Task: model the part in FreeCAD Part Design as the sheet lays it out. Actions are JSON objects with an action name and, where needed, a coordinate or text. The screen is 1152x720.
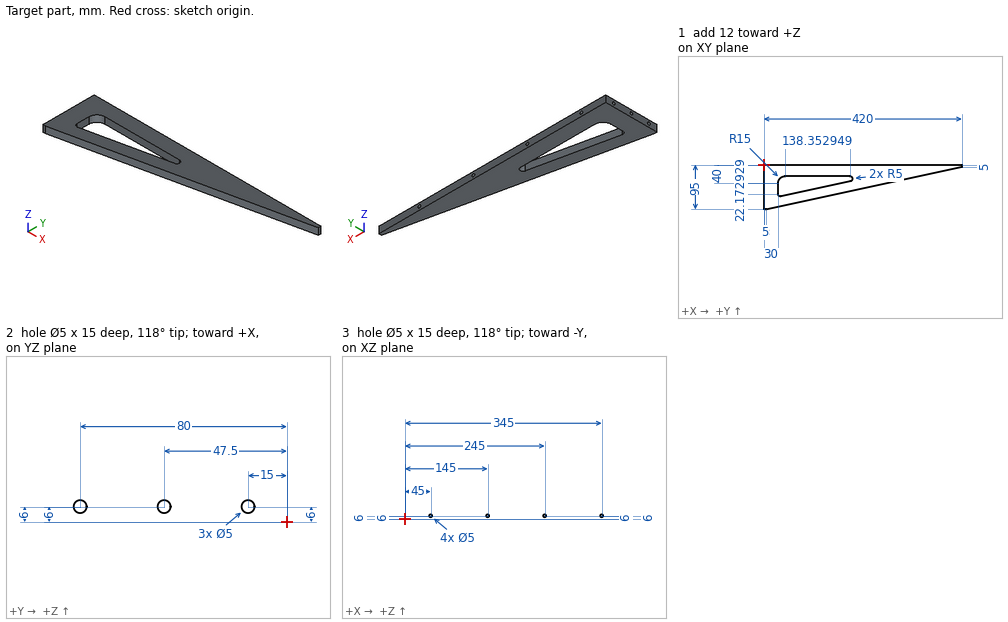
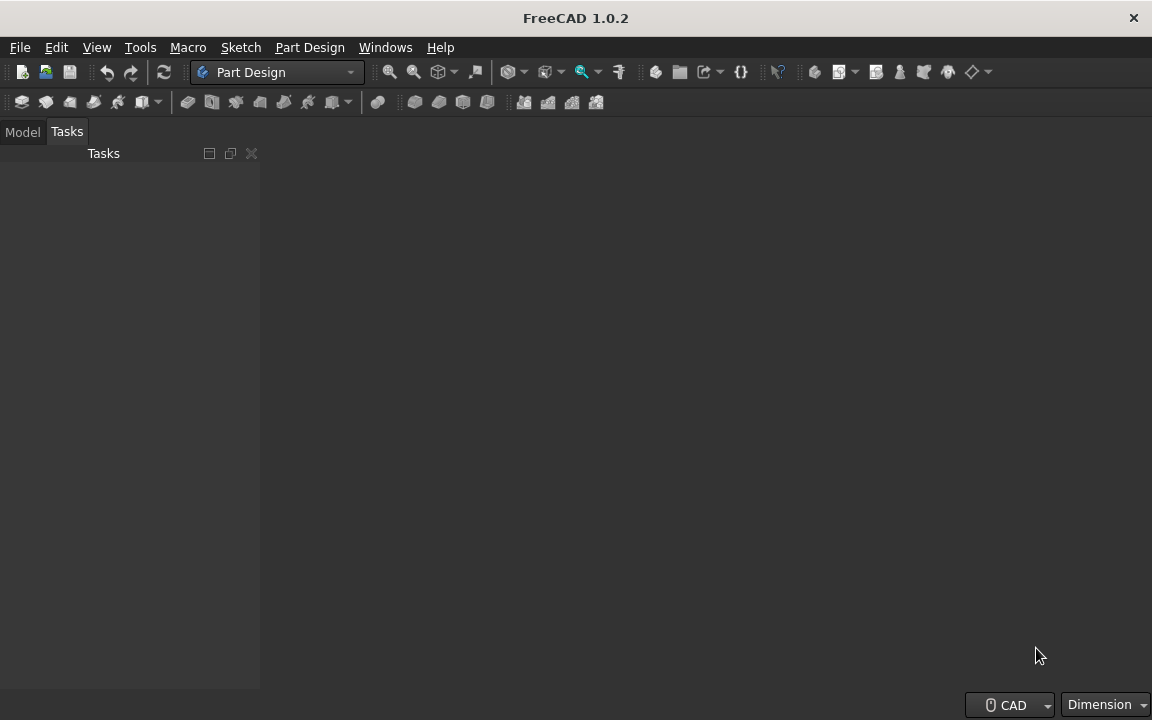
{"action": "left_click", "coordinate": [22, 72]}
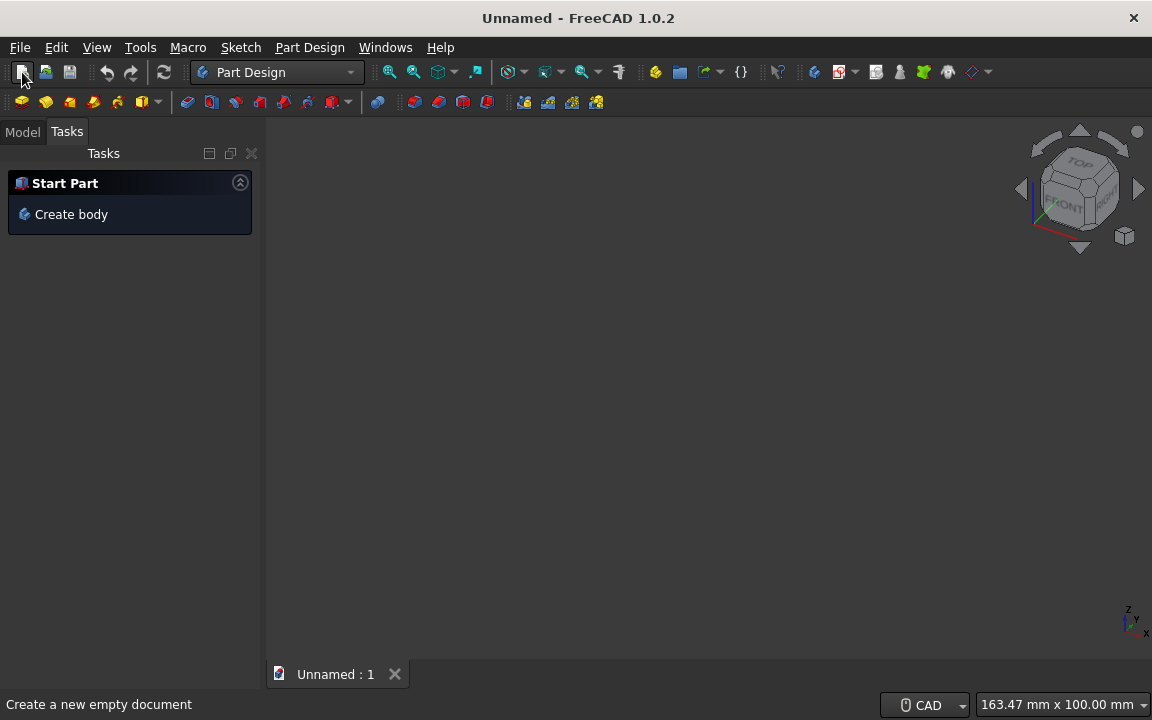
{"action": "left_click", "coordinate": [840, 72]}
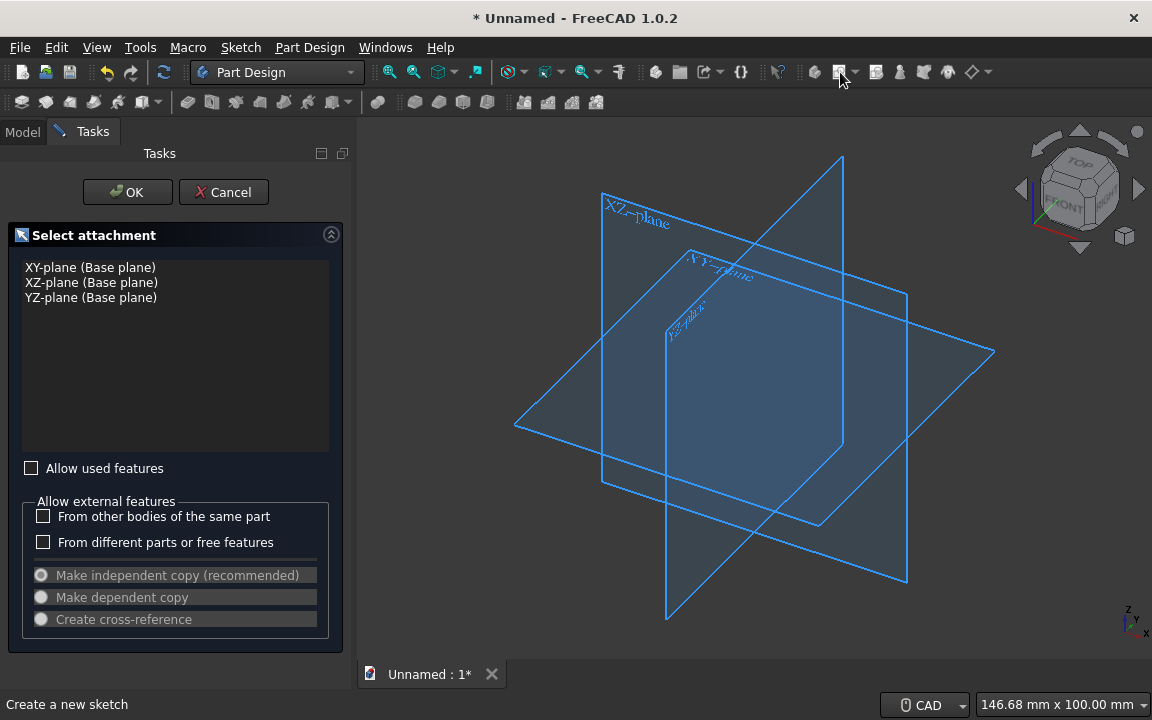
{"action": "left_click", "coordinate": [82, 268]}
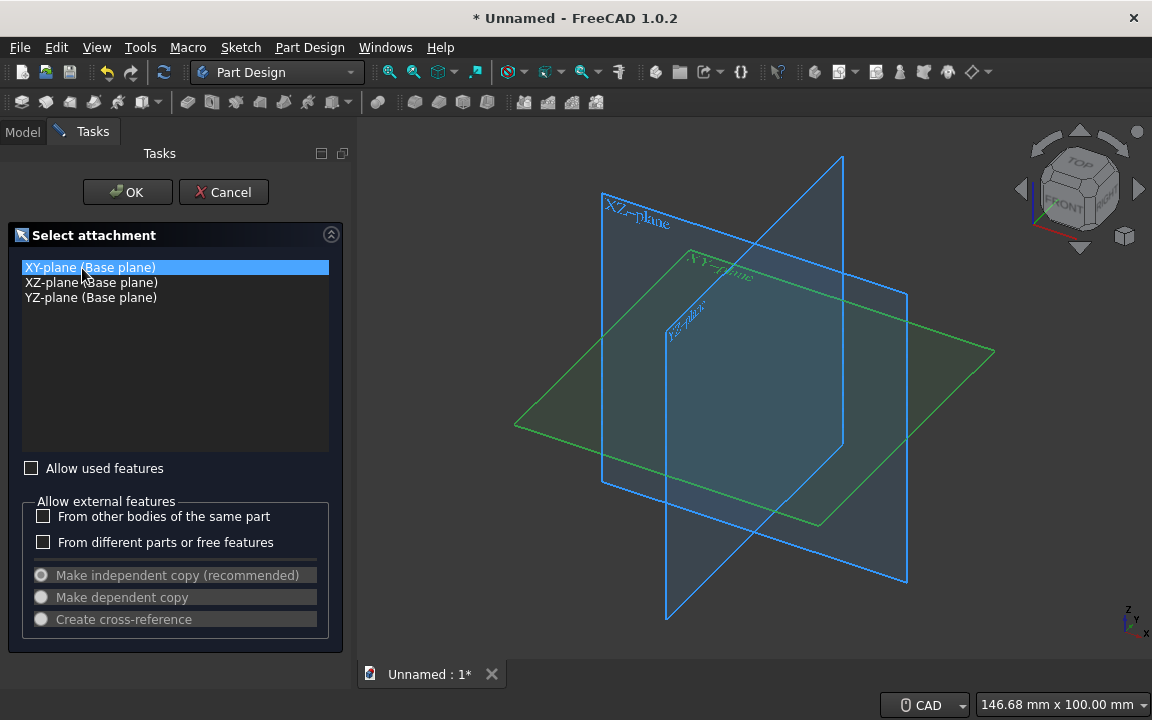
{"action": "left_click", "coordinate": [128, 192]}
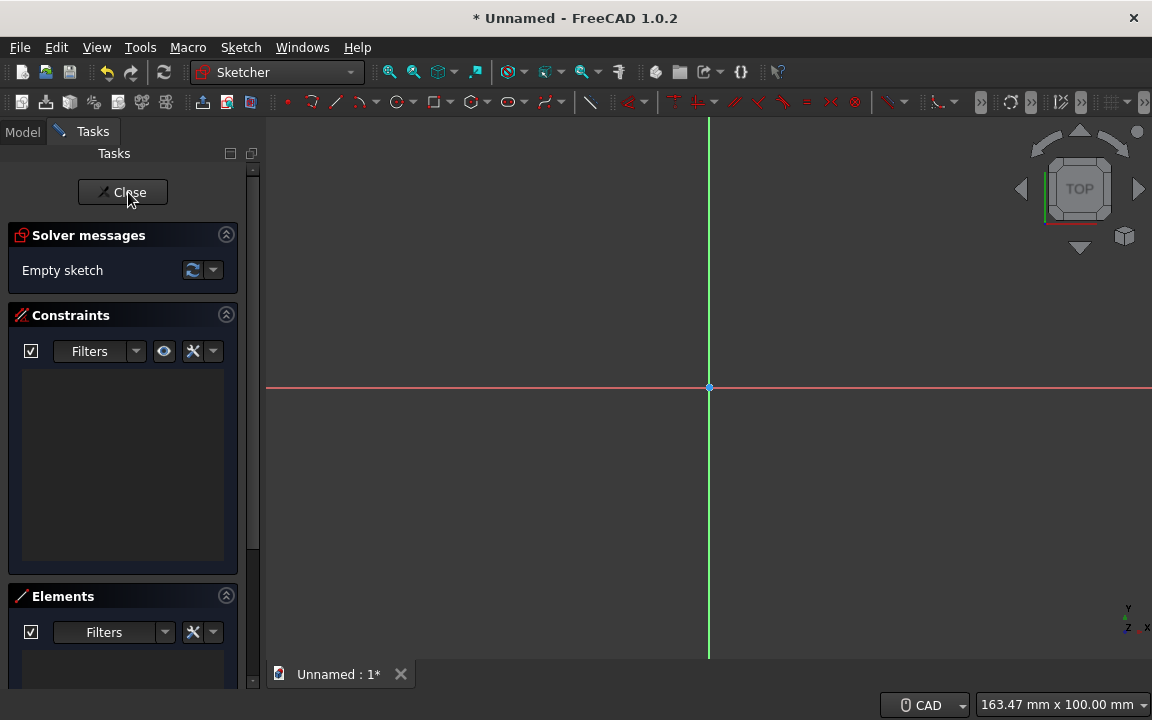
{"action": "scroll", "coordinate": [335, 323], "scroll_direction": "down", "scroll_amount": 8}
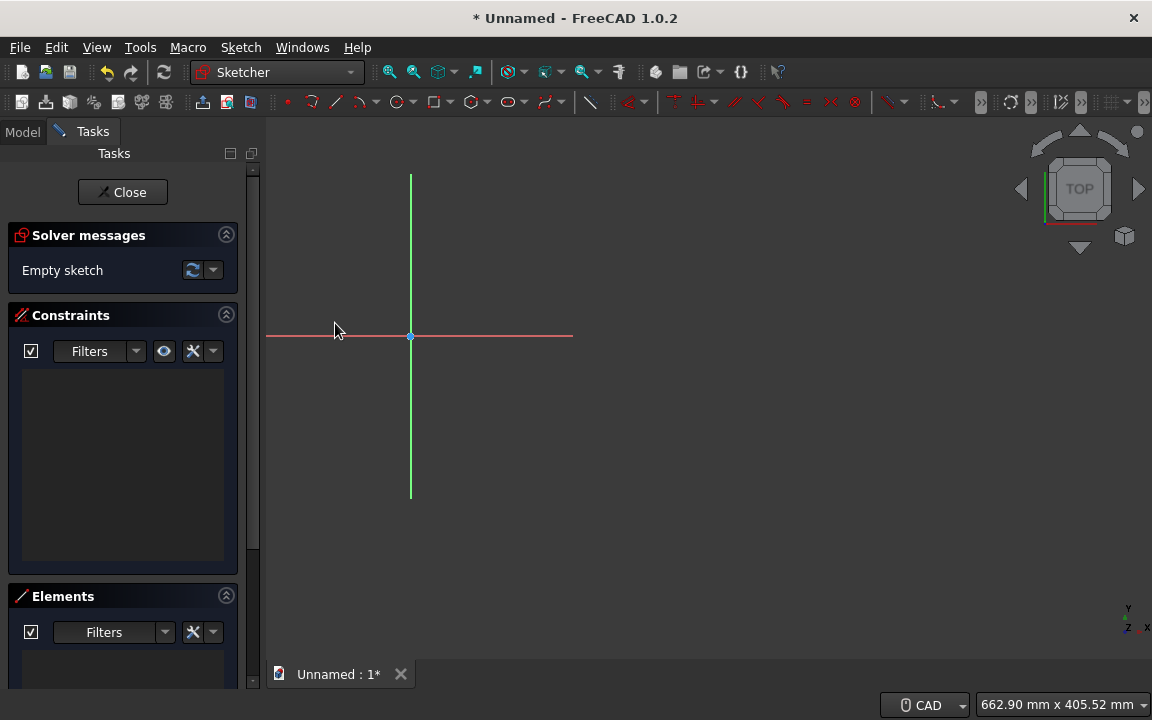
{"action": "left_click", "coordinate": [312, 102]}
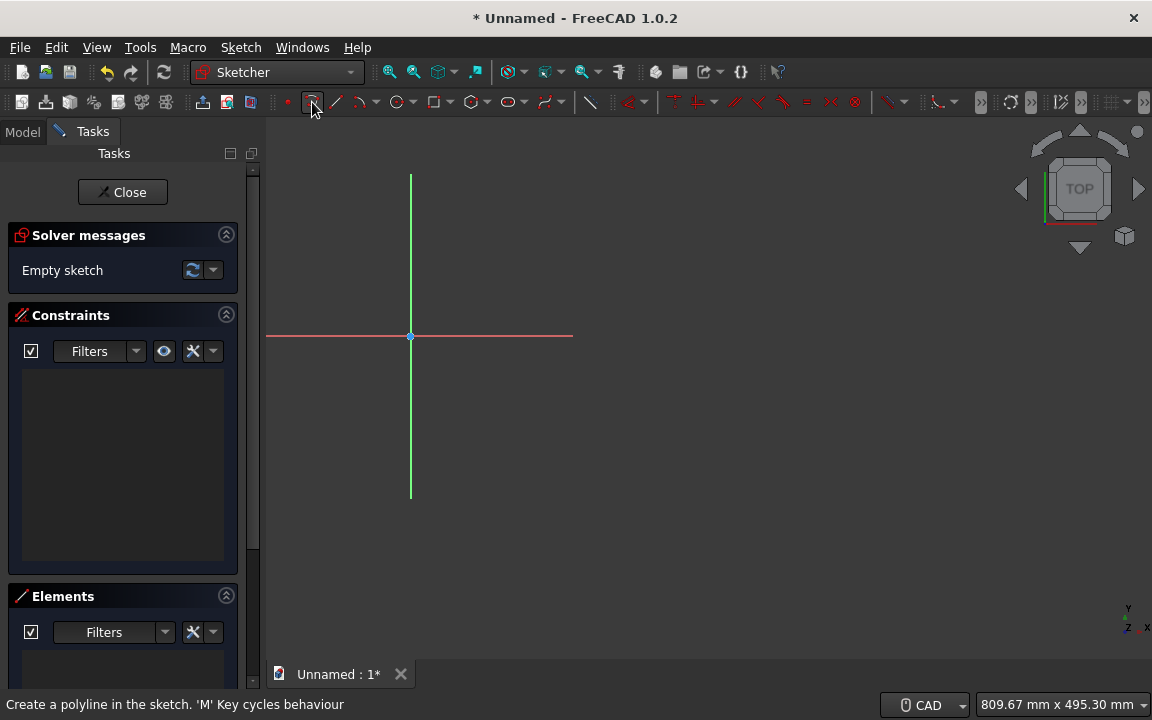
{"action": "left_click", "coordinate": [411, 336]}
{"action": "left_click", "coordinate": [420, 440]}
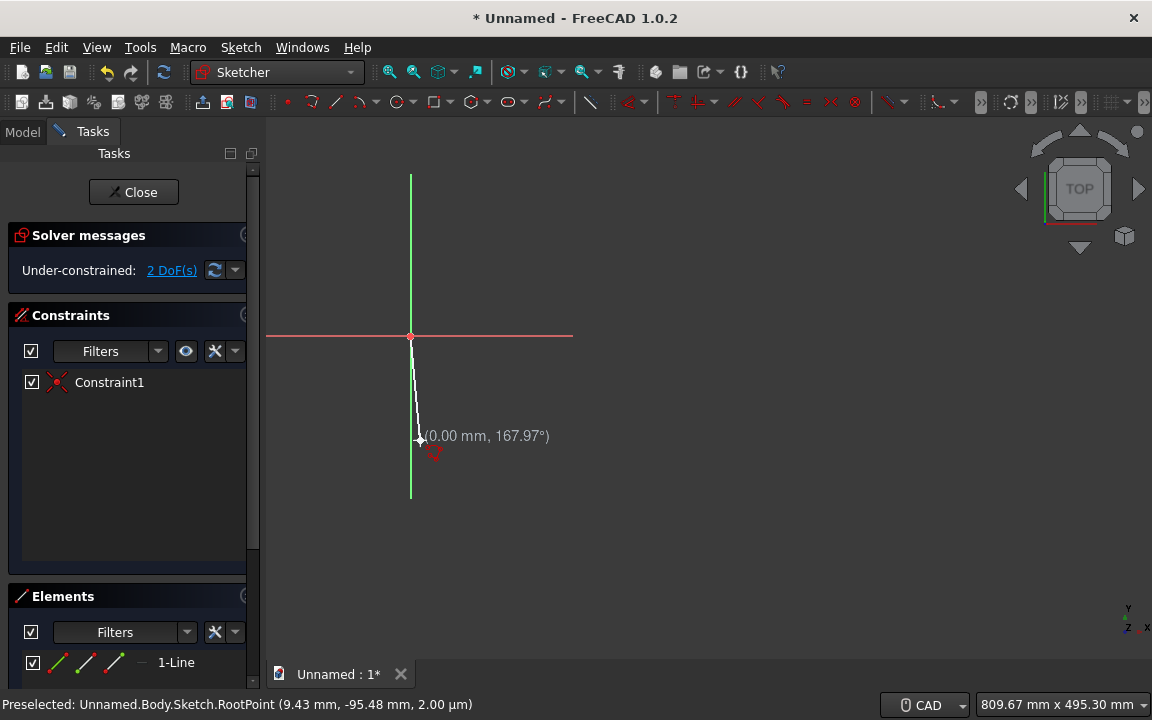
{"action": "scroll", "coordinate": [416, 440], "scroll_direction": "up", "scroll_amount": 6}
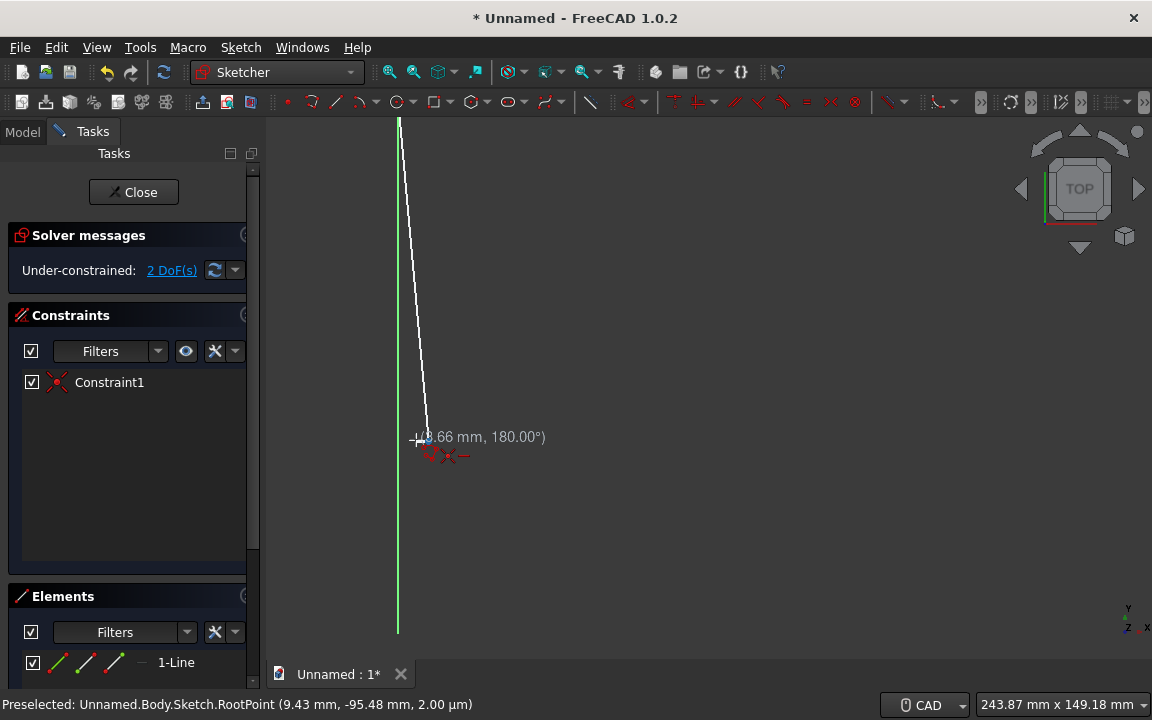
{"action": "left_click", "coordinate": [416, 439]}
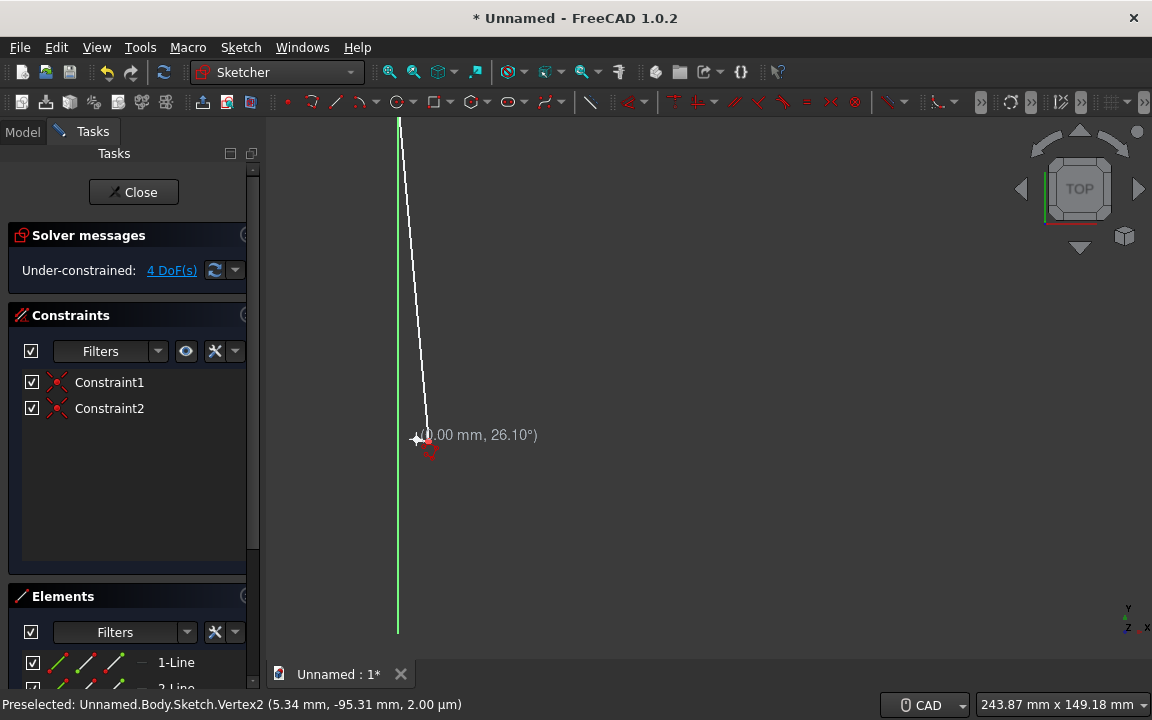
{"action": "scroll", "coordinate": [416, 440], "scroll_direction": "down", "scroll_amount": 6}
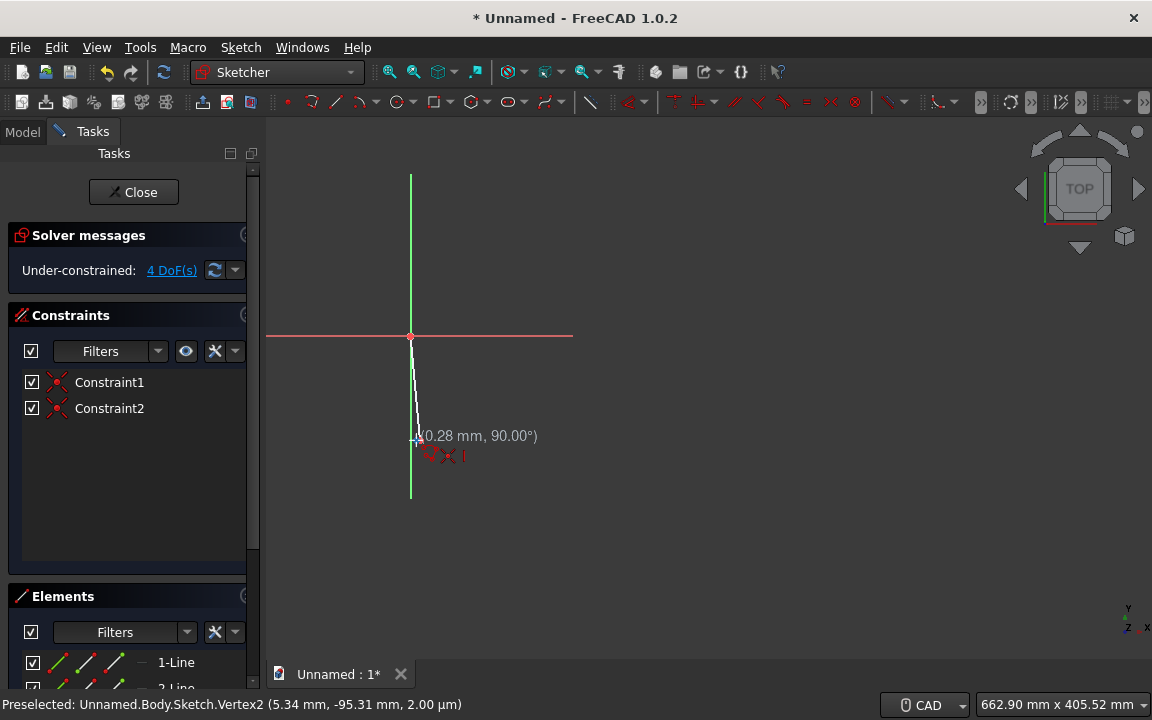
{"action": "scroll", "coordinate": [870, 342], "scroll_direction": "up", "scroll_amount": 6}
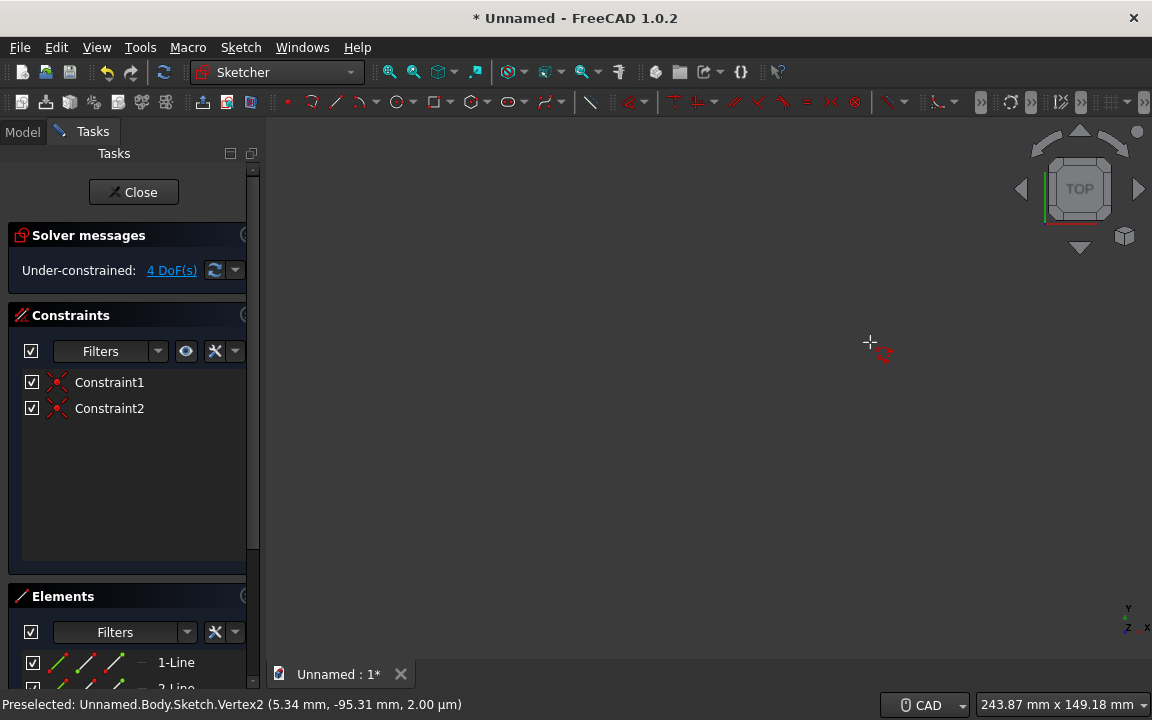
{"action": "left_click", "coordinate": [869, 341]}
{"action": "left_click", "coordinate": [869, 332]}